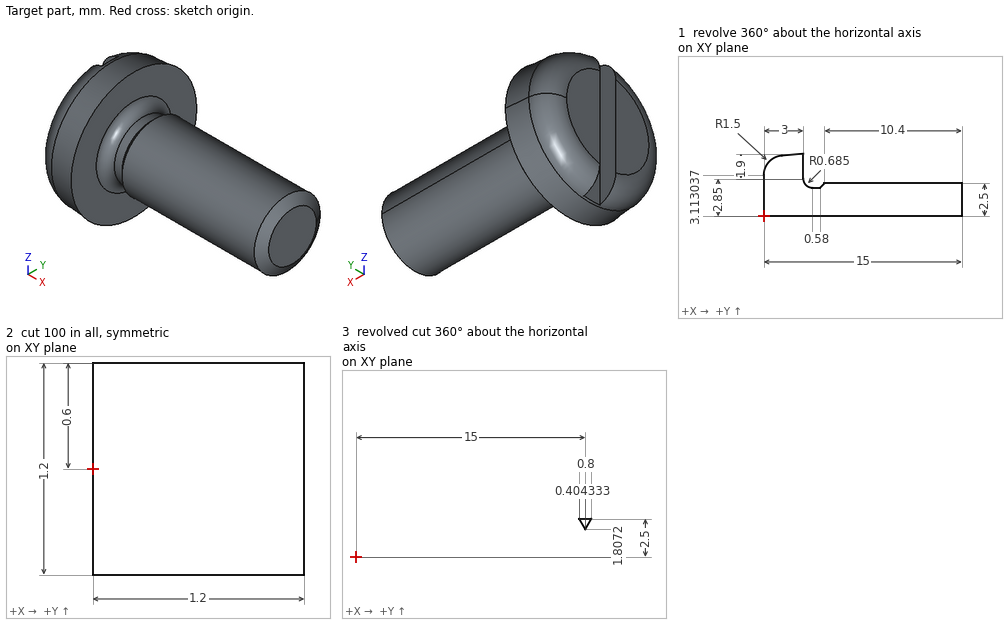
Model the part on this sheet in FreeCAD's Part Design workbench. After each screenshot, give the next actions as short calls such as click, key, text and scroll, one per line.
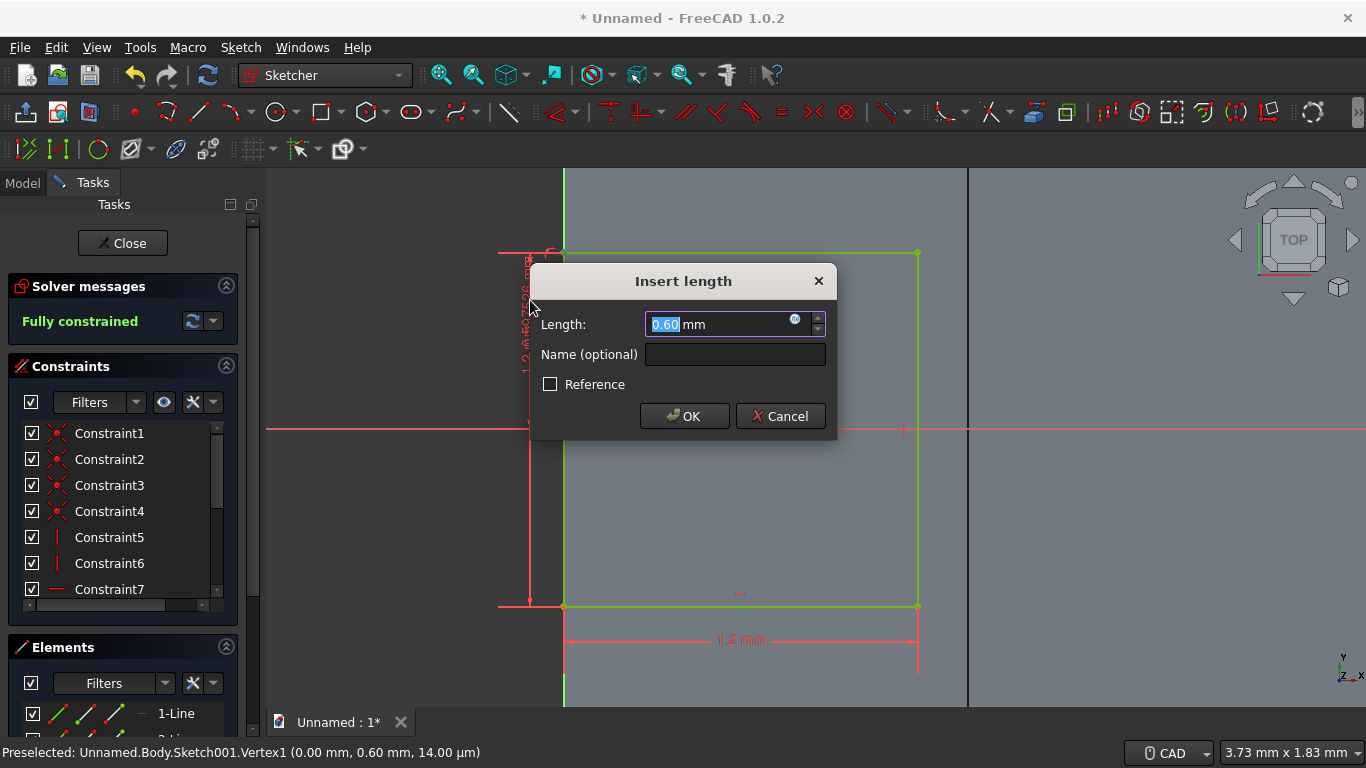
text(0.6)
key(Return)
key(Escape)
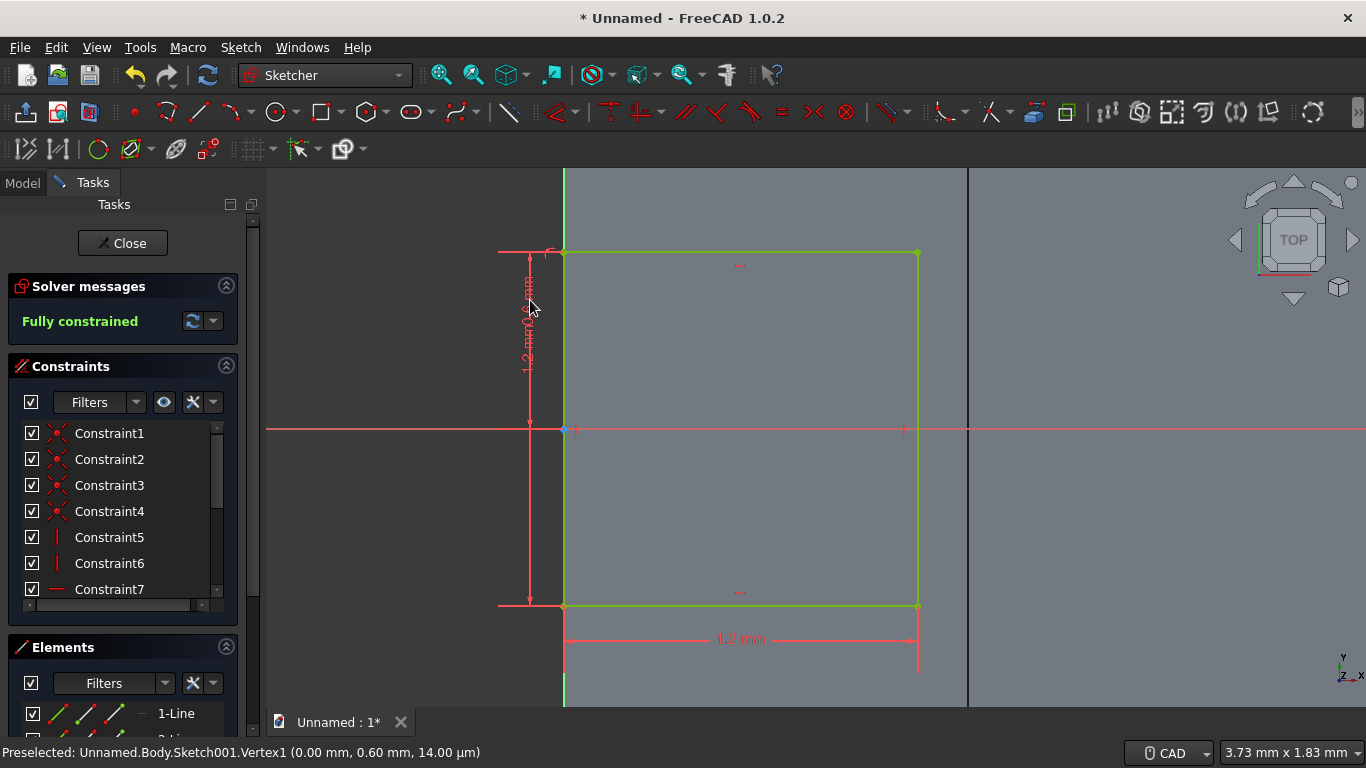
click(123, 243)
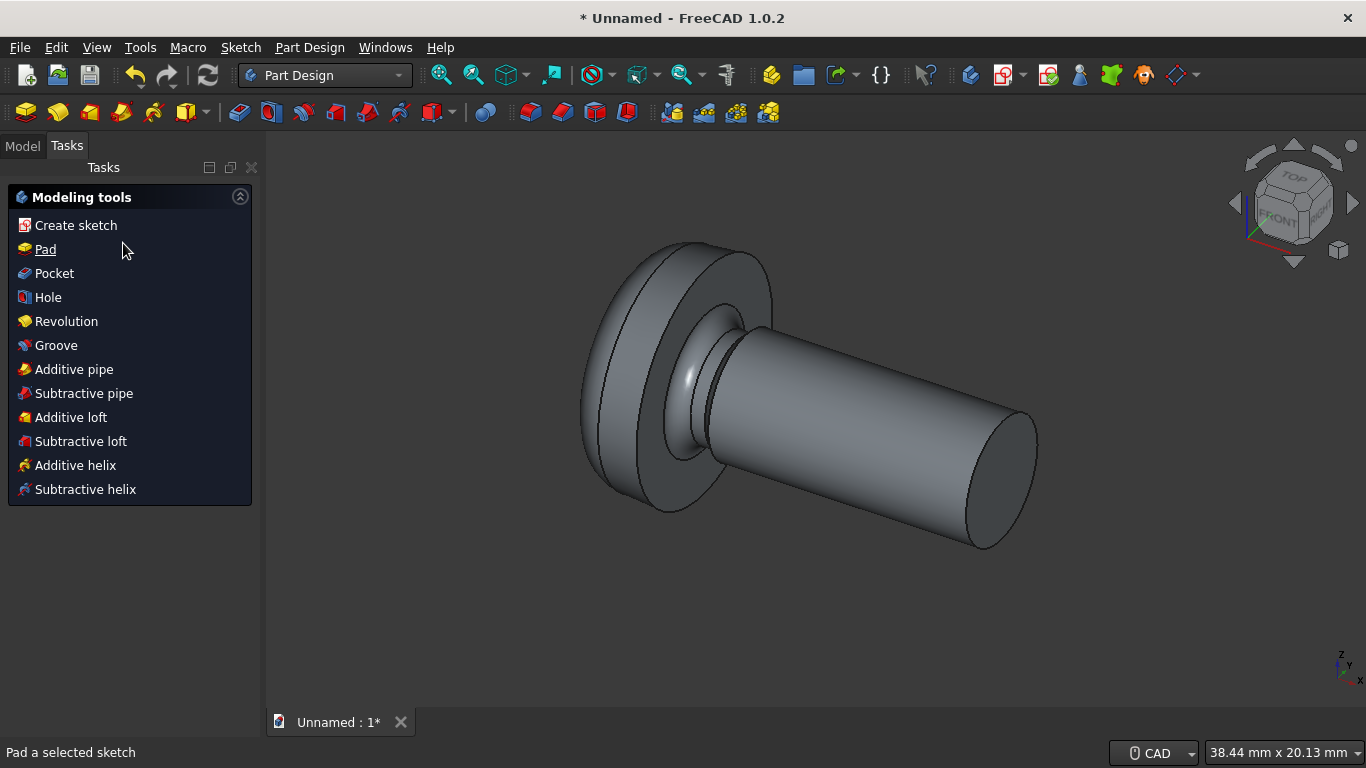
click(240, 112)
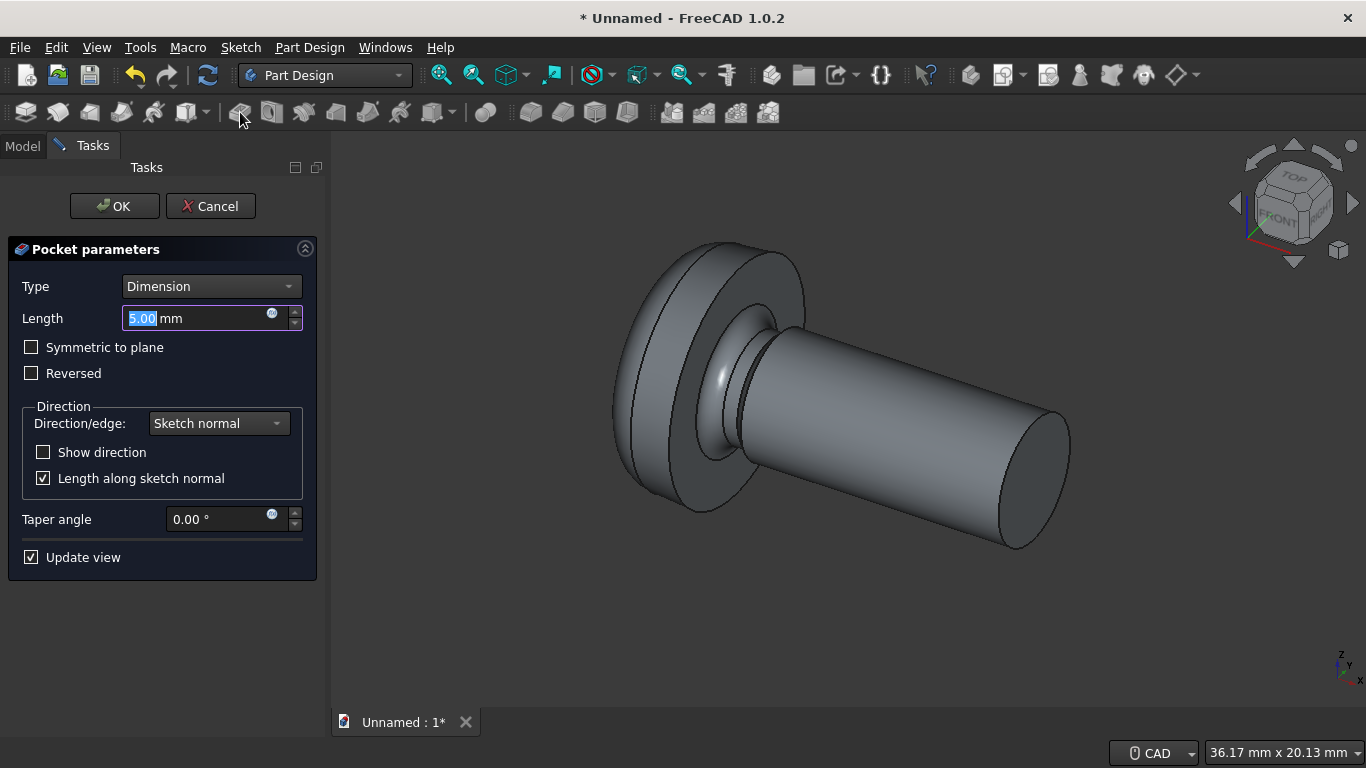
text(100)
key(Tab)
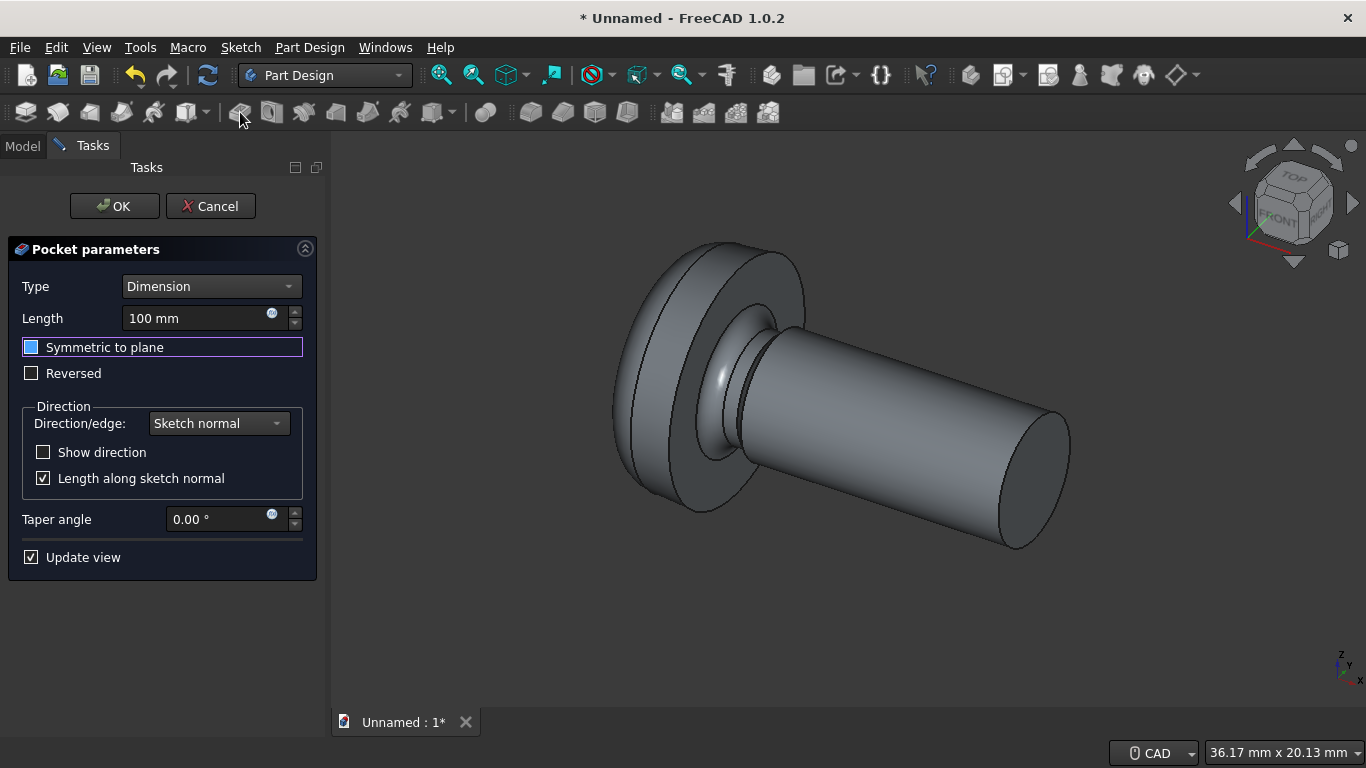
click(30, 347)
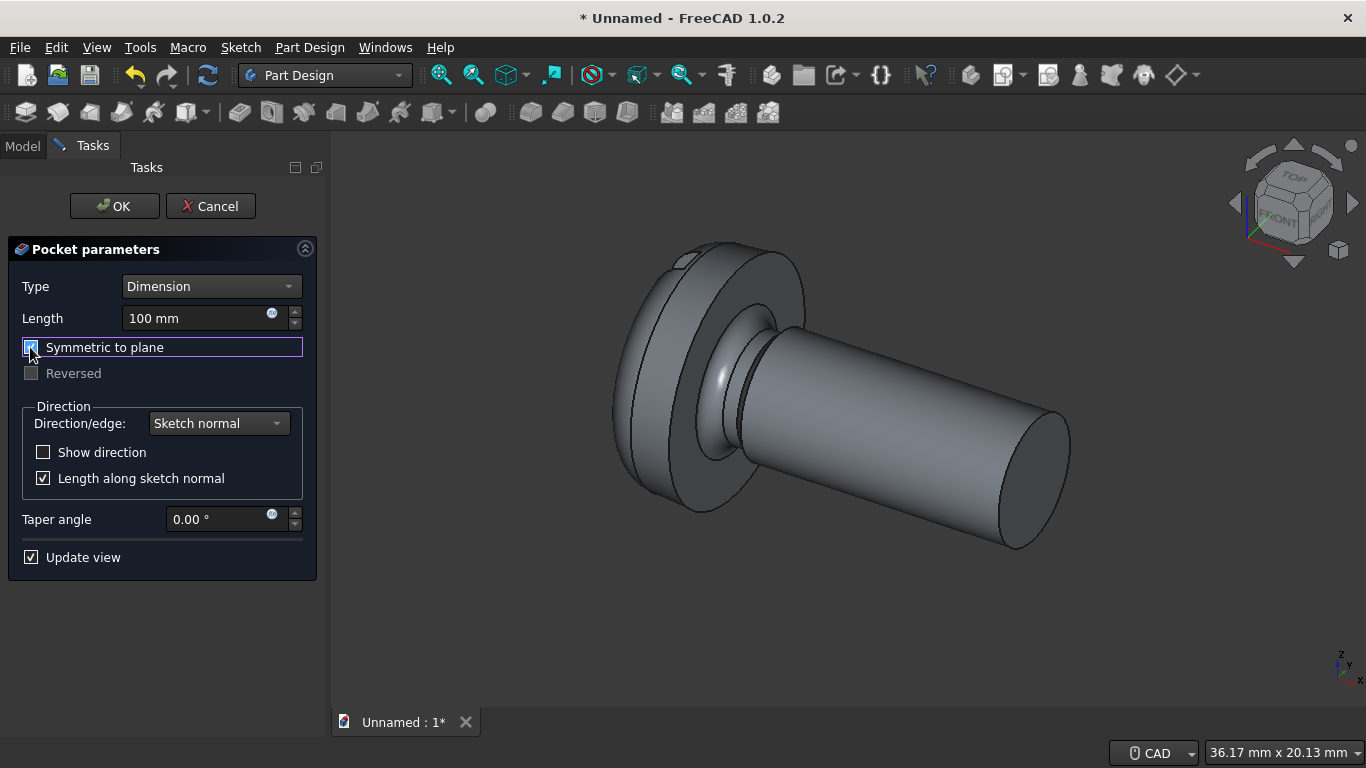
click(115, 206)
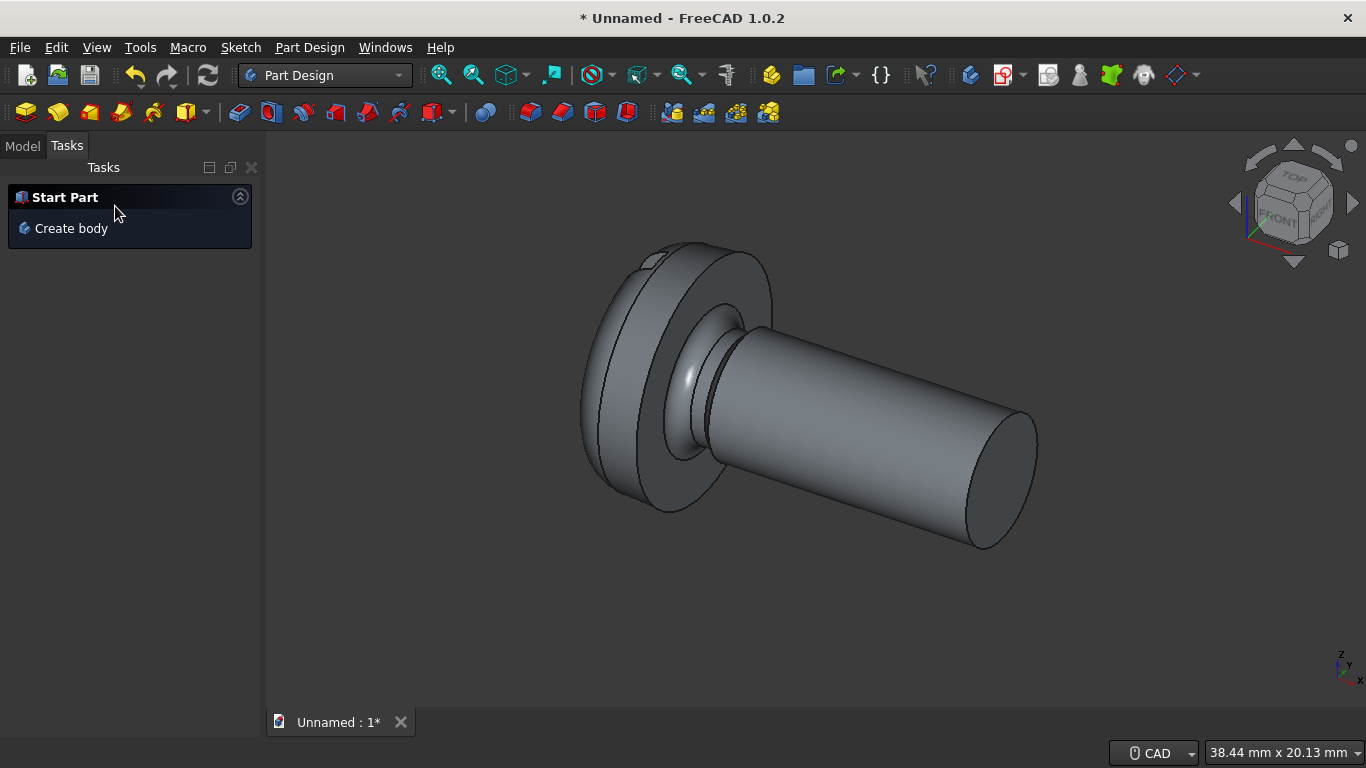
click(1004, 76)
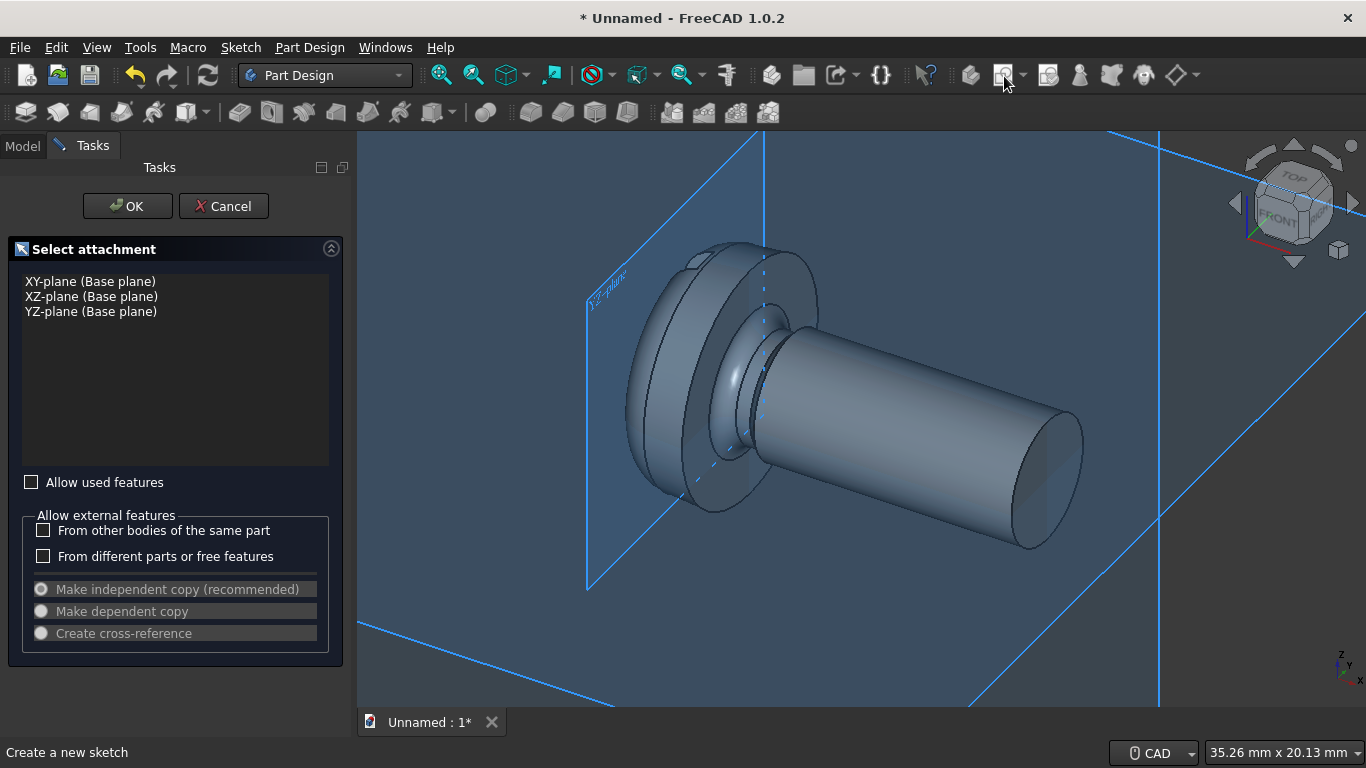
click(82, 282)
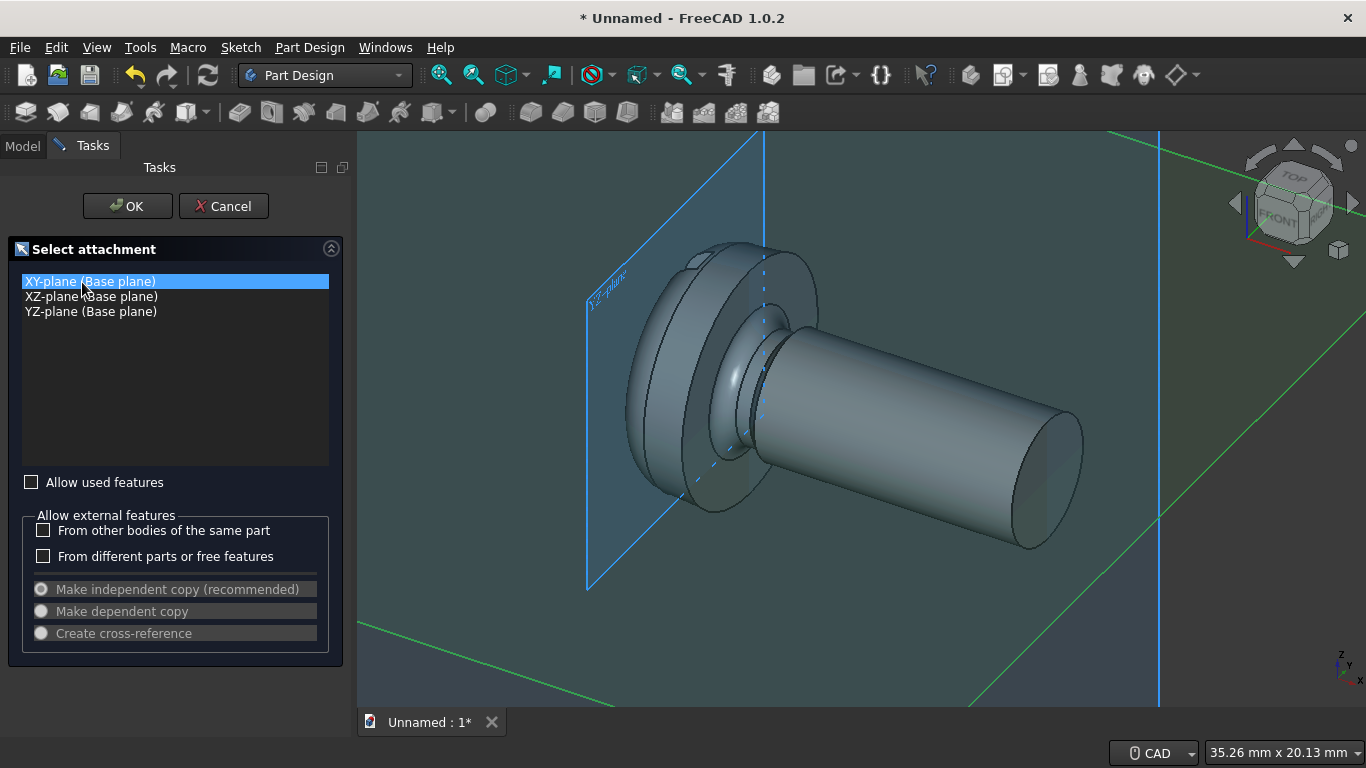
click(128, 206)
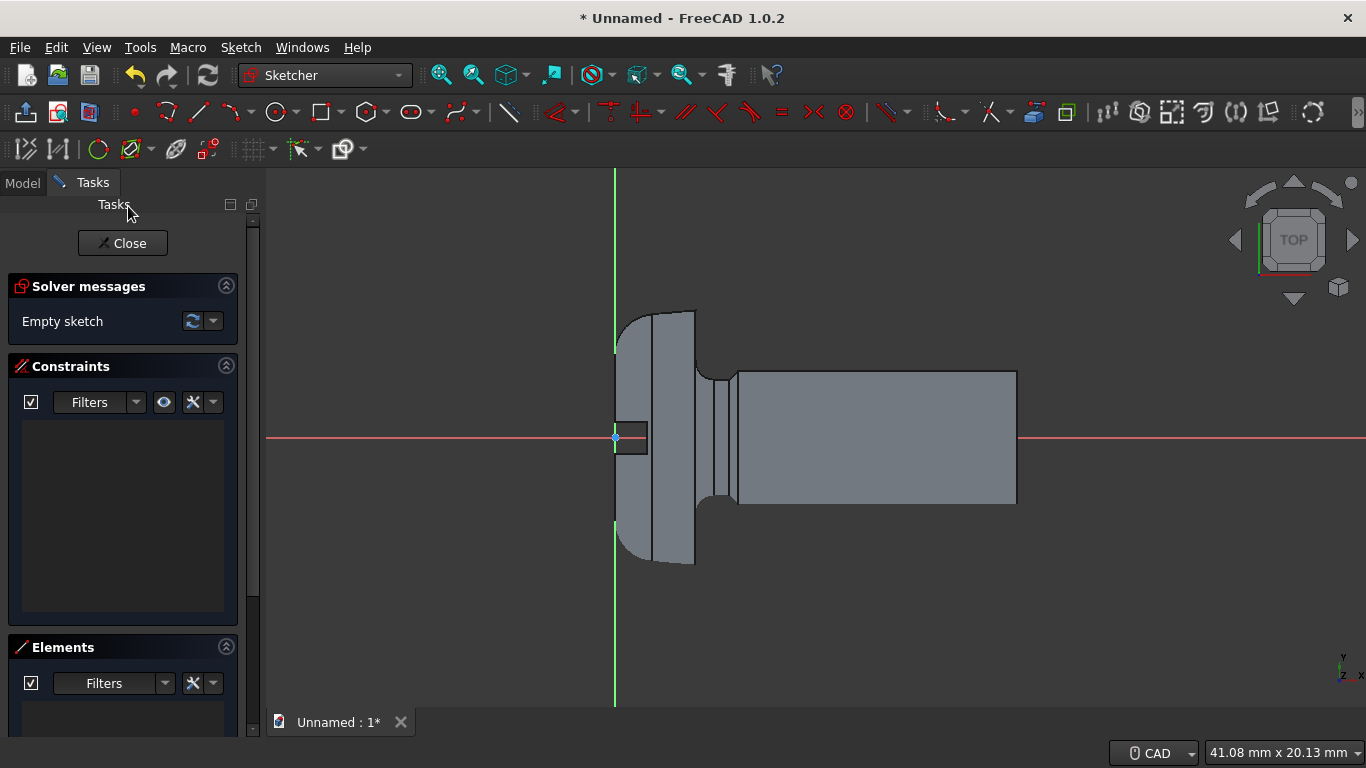
click(90, 112)